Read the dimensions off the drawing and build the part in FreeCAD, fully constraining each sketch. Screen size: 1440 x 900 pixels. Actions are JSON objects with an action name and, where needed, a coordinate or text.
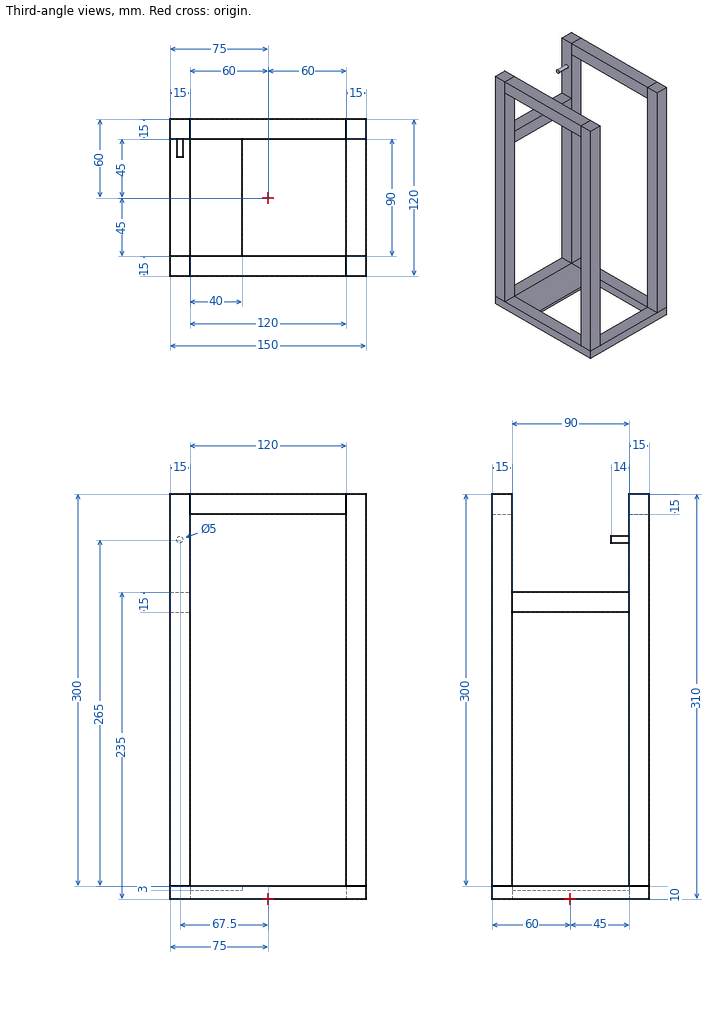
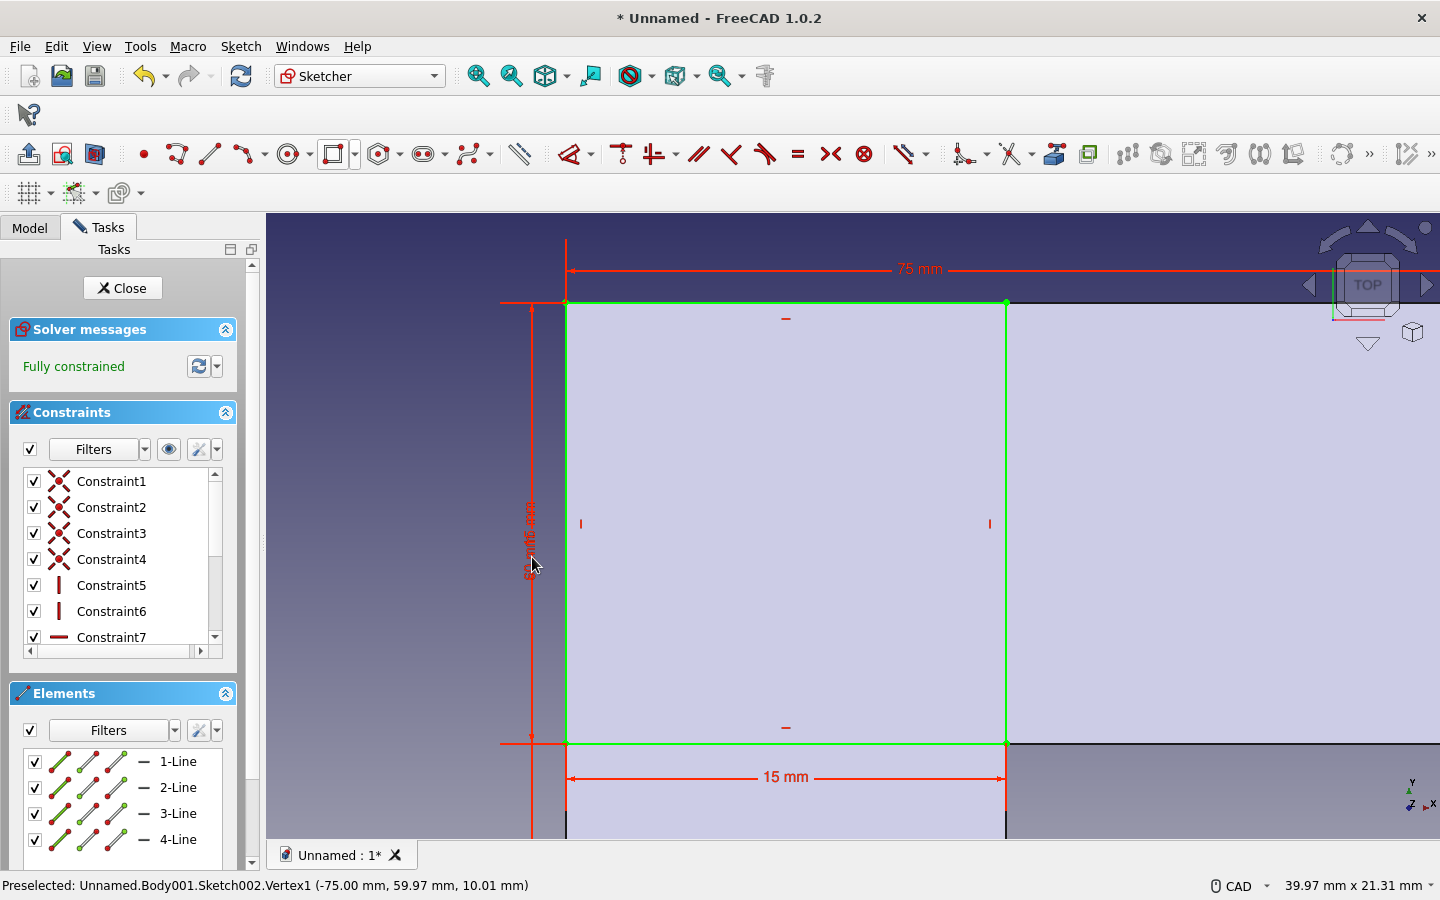
{"action": "left_click", "coordinate": [123, 288]}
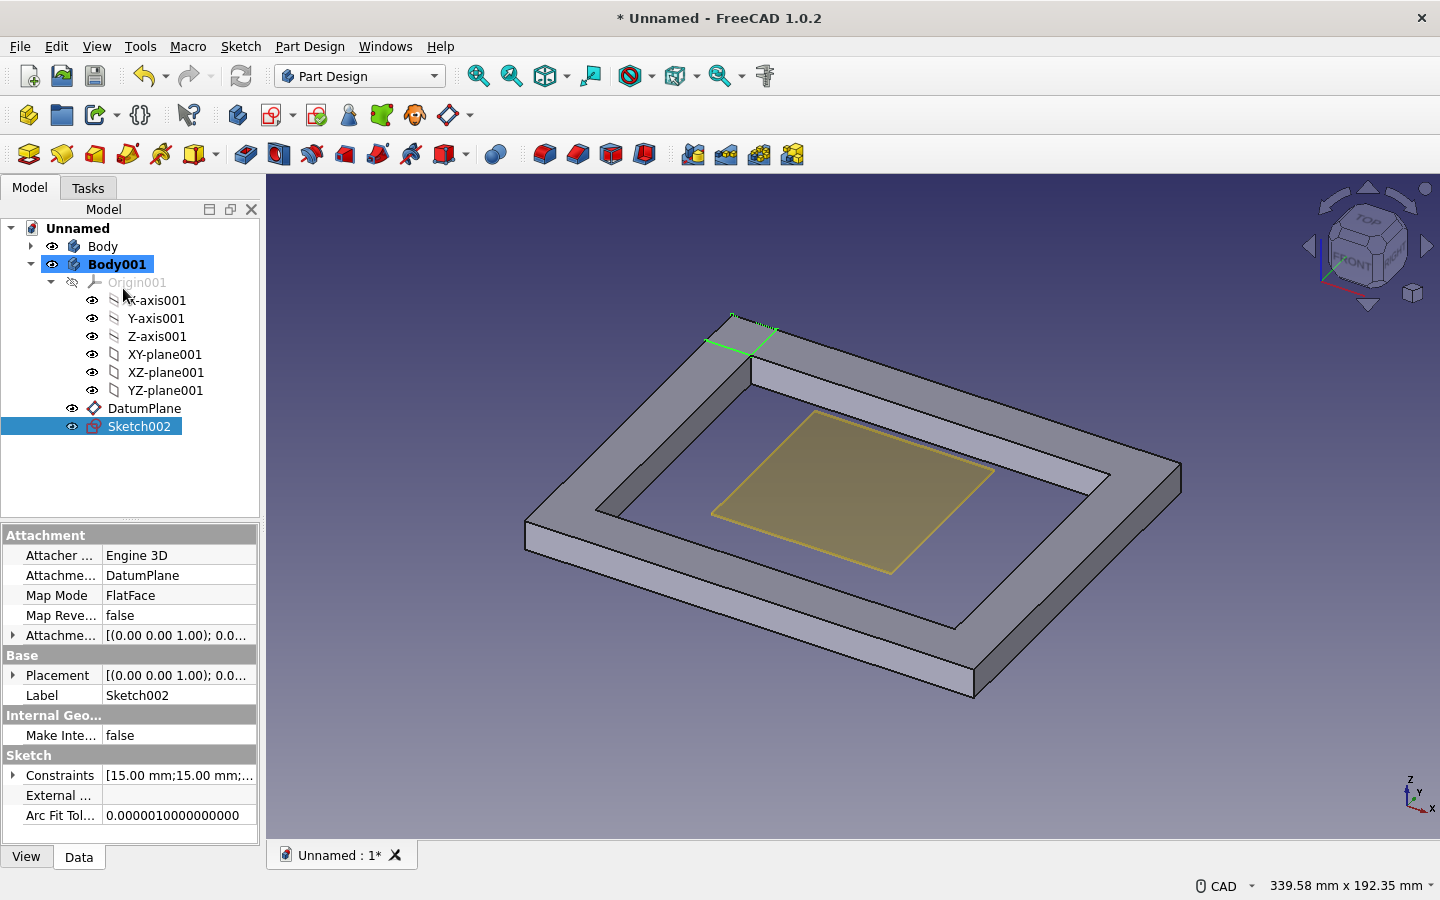
{"action": "left_click", "coordinate": [29, 154]}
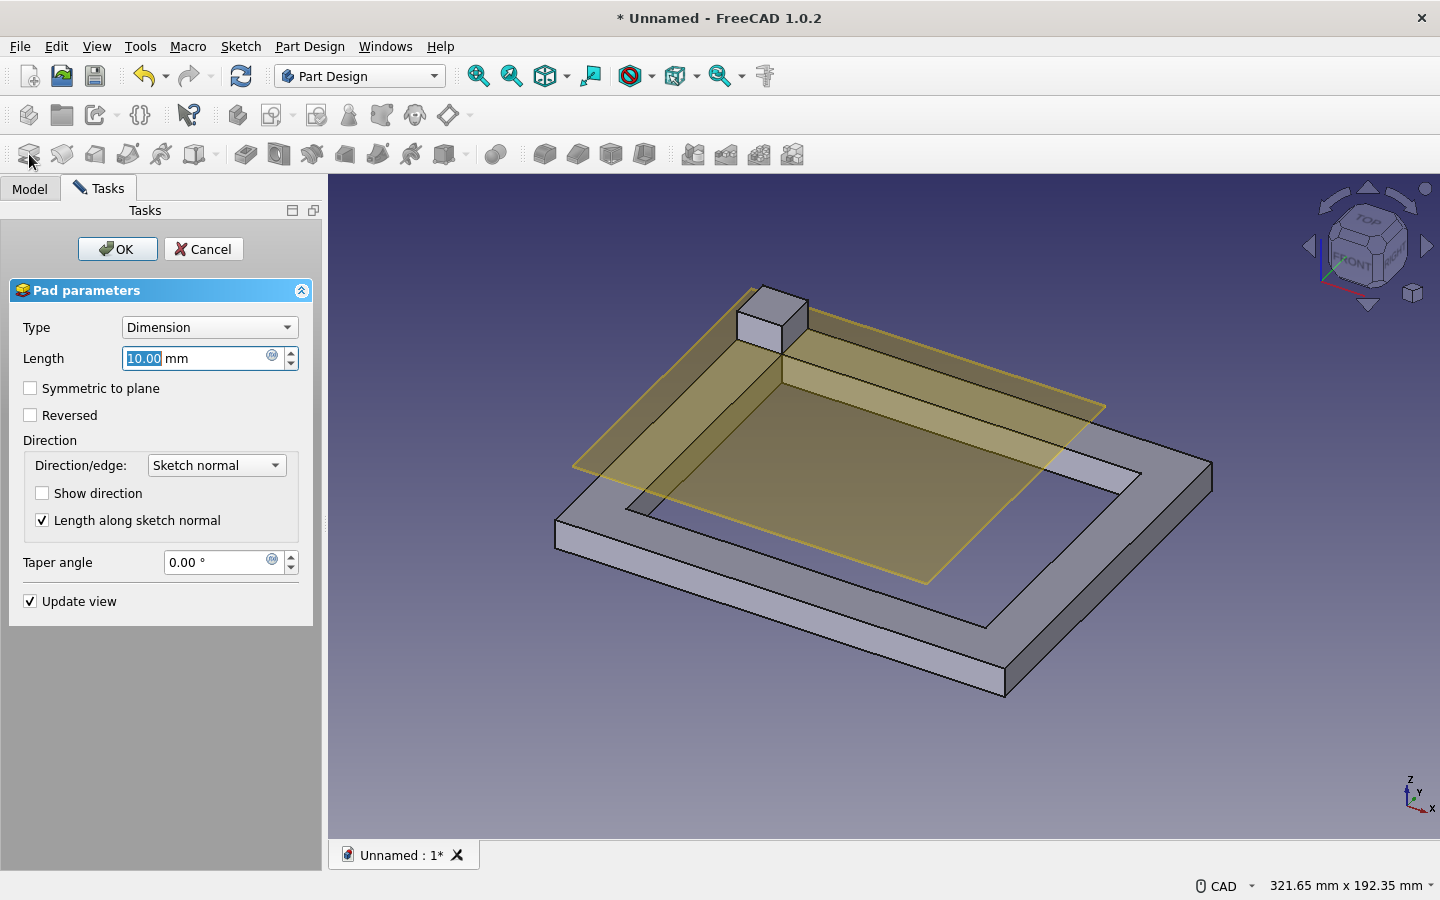
{"action": "type", "text": "300"}
{"action": "key", "text": "Tab"}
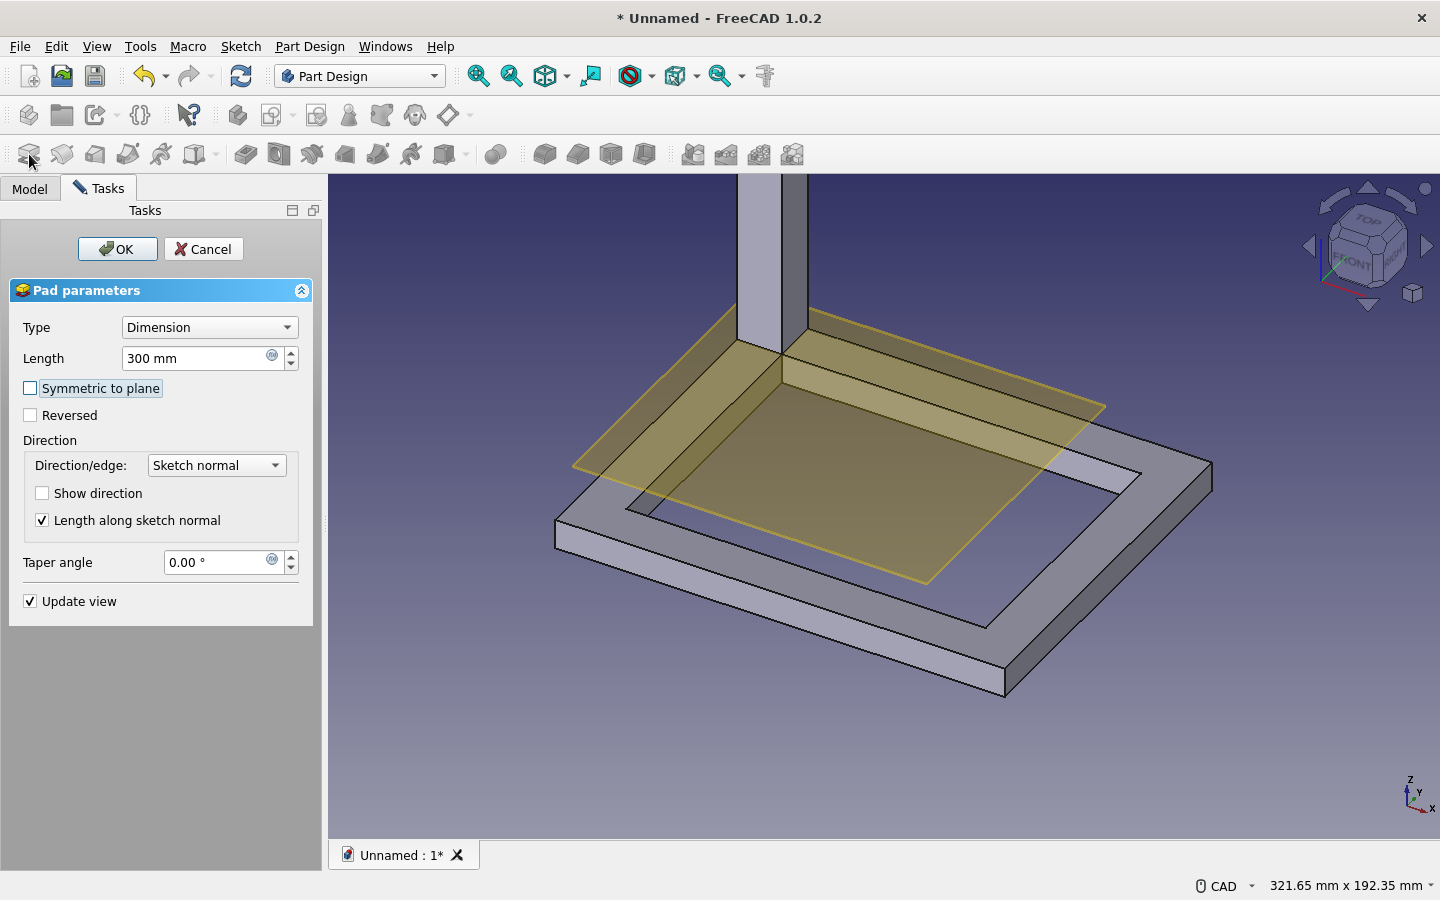
{"action": "left_click", "coordinate": [118, 249]}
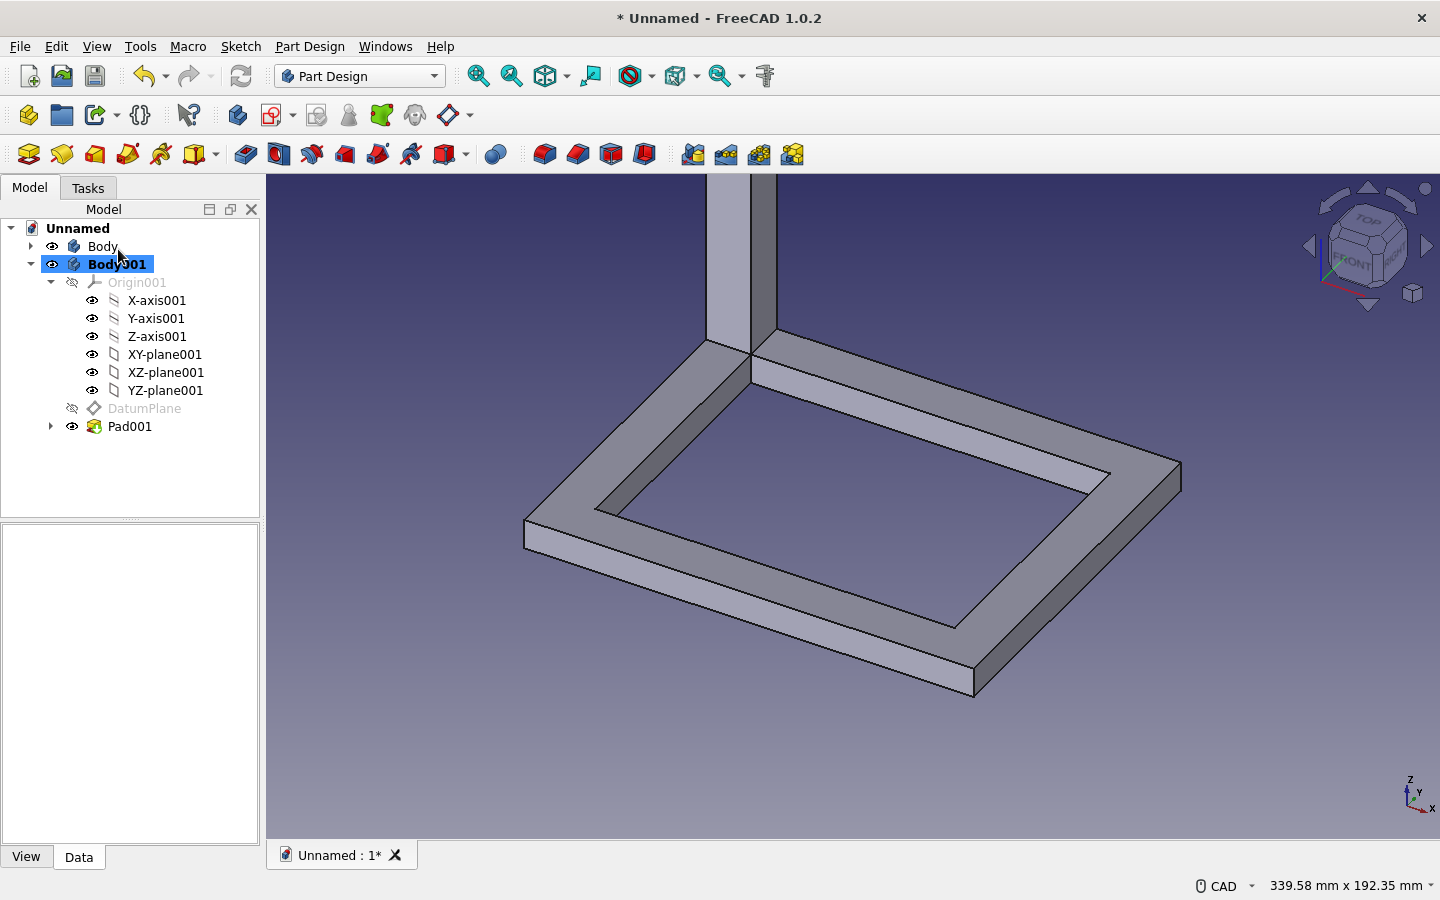
{"action": "left_click", "coordinate": [479, 76]}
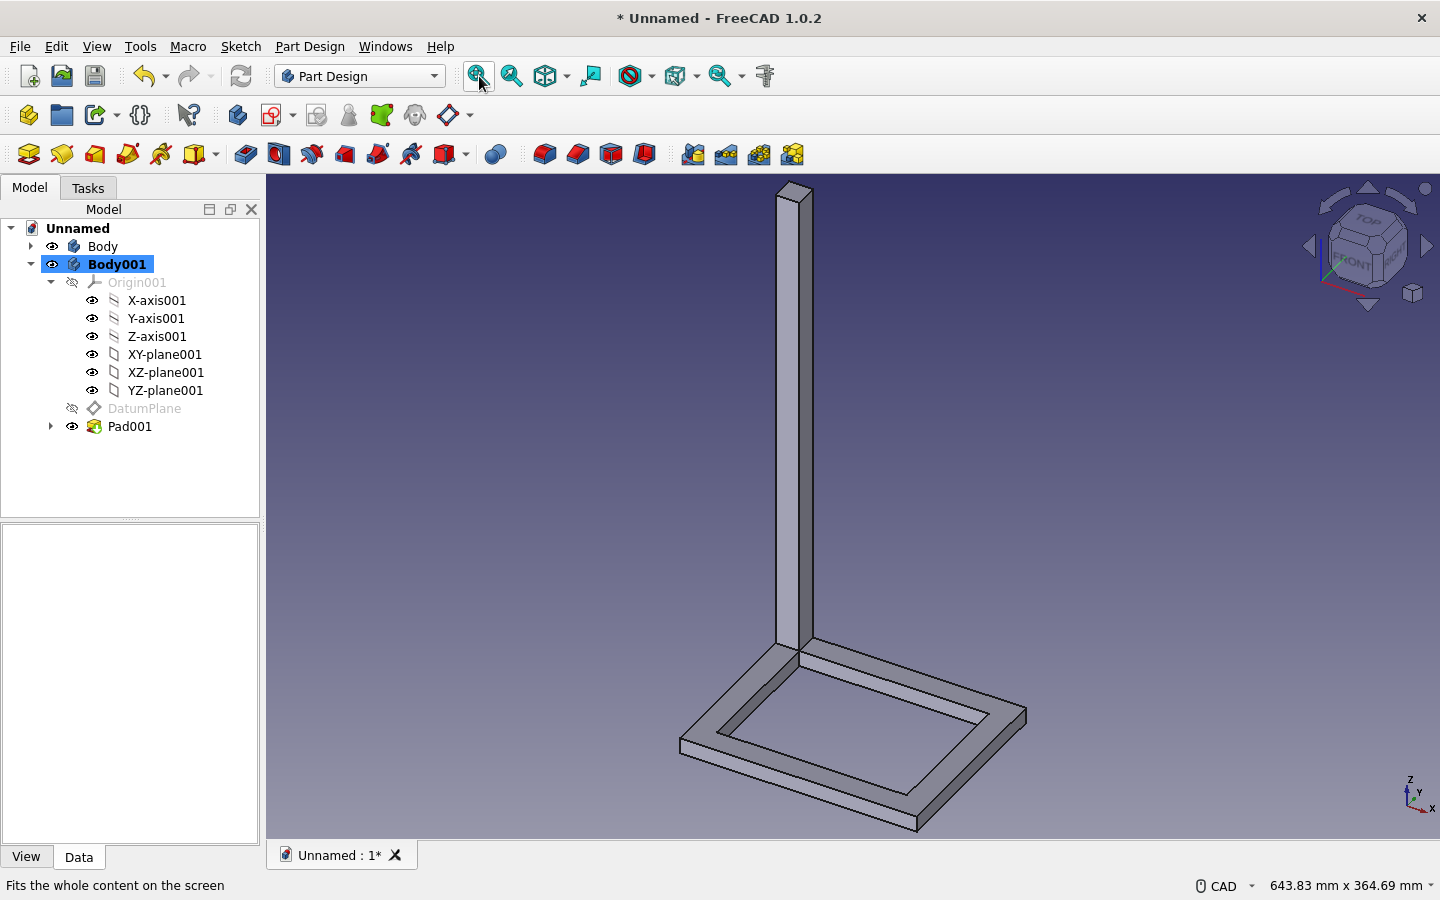
{"action": "left_click", "coordinate": [787, 230]}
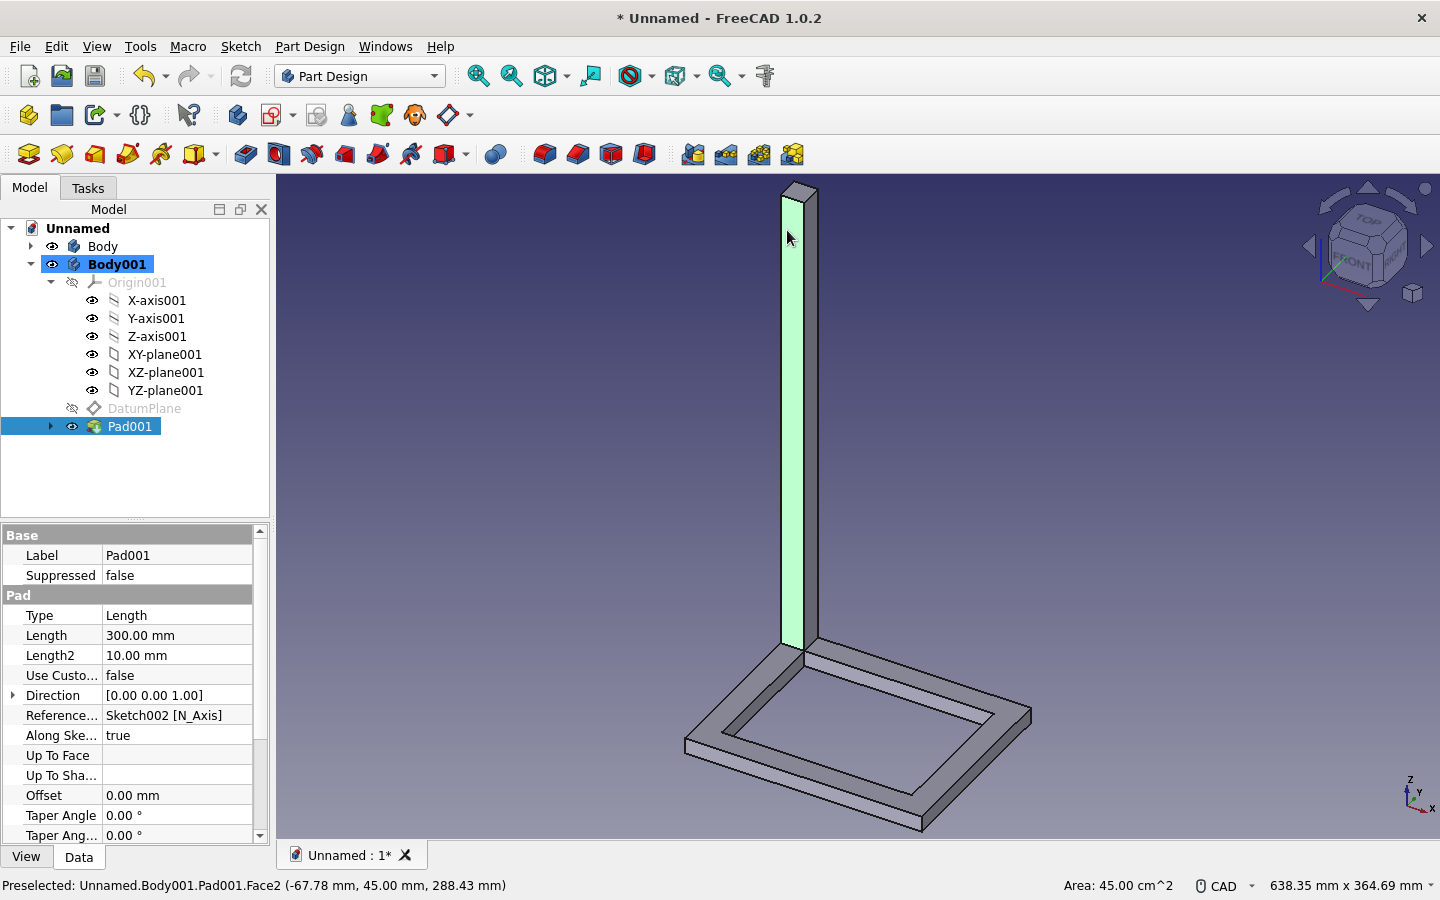
{"action": "left_click", "coordinate": [270, 116]}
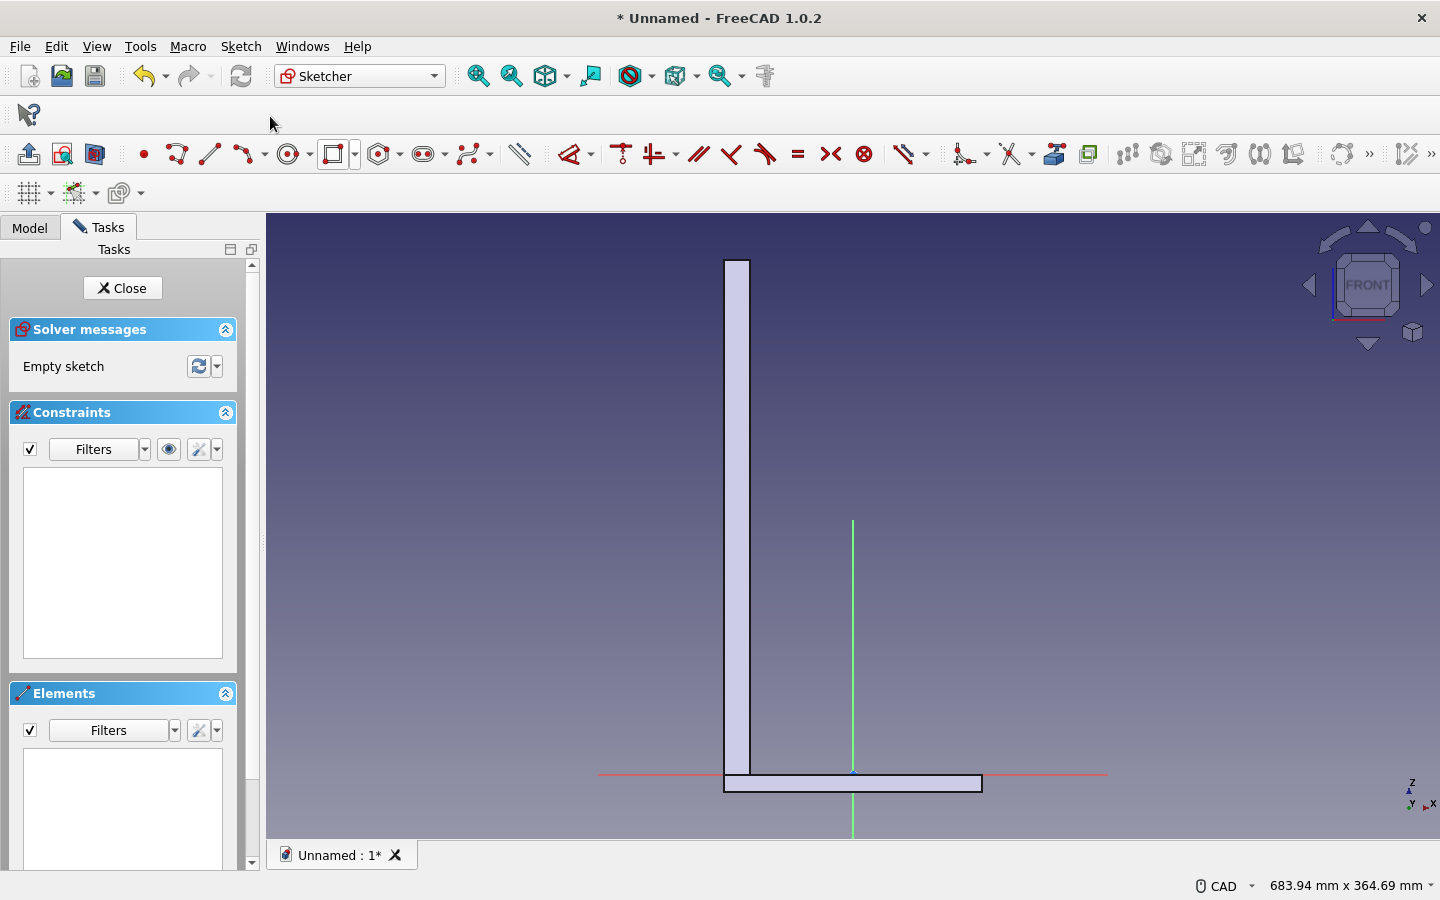
{"action": "scroll", "coordinate": [735, 309], "scroll_direction": "up", "scroll_amount": 15}